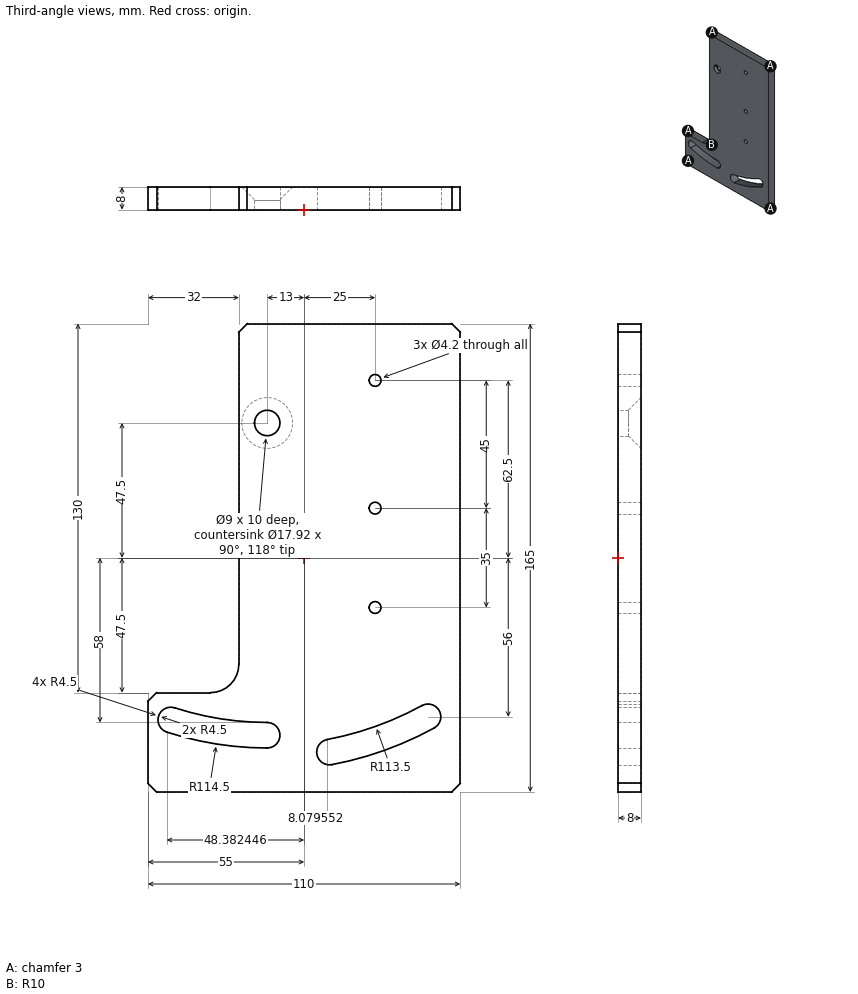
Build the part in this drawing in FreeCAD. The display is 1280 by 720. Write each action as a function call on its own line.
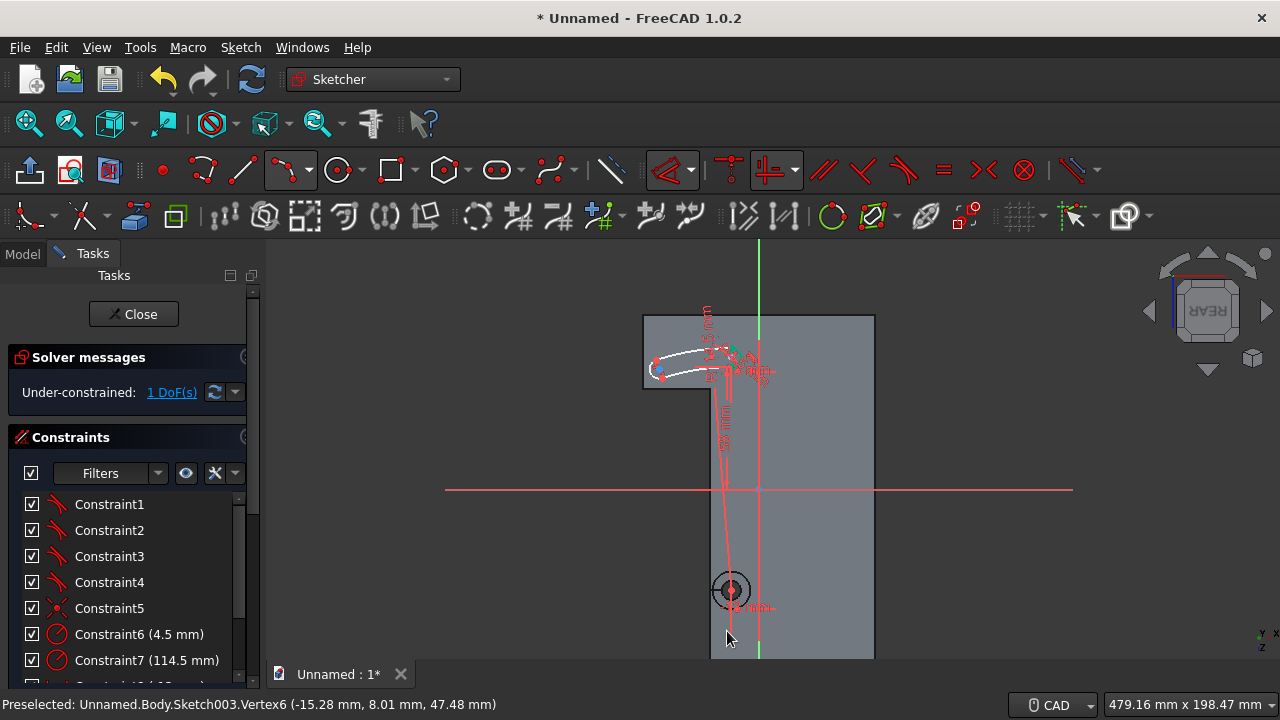
scroll(705, 383, up, 3)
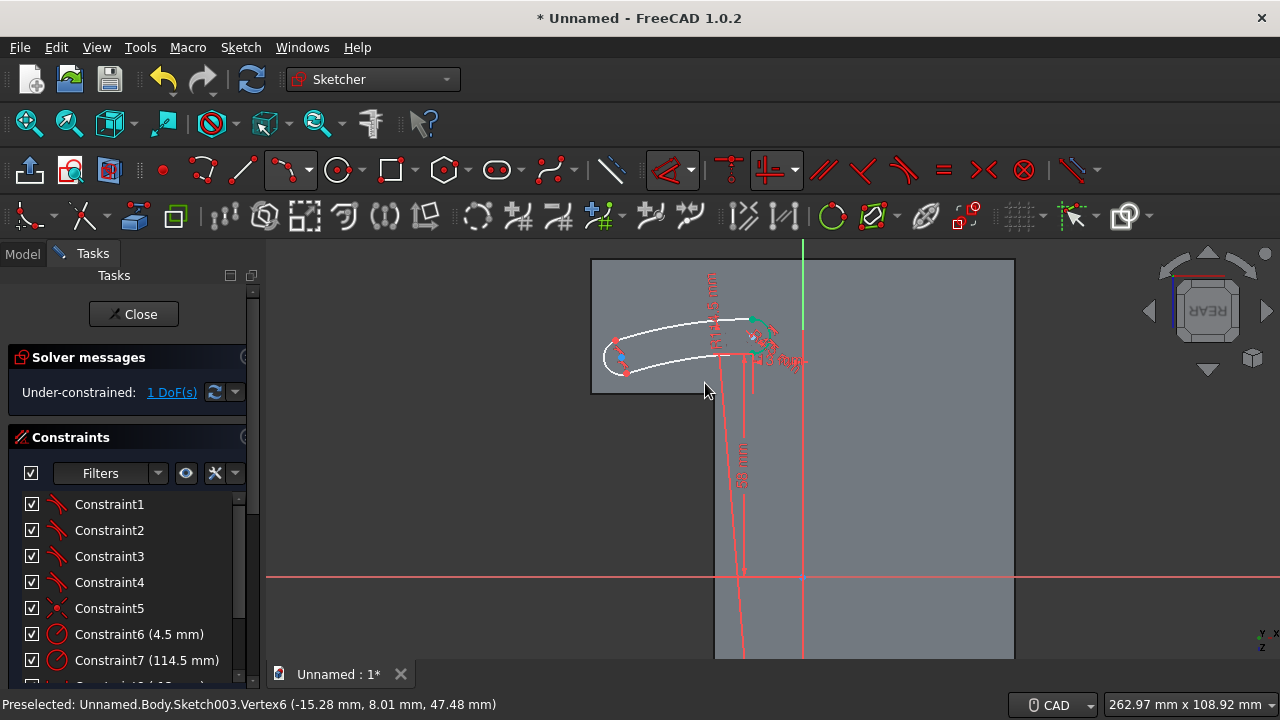
click(616, 341)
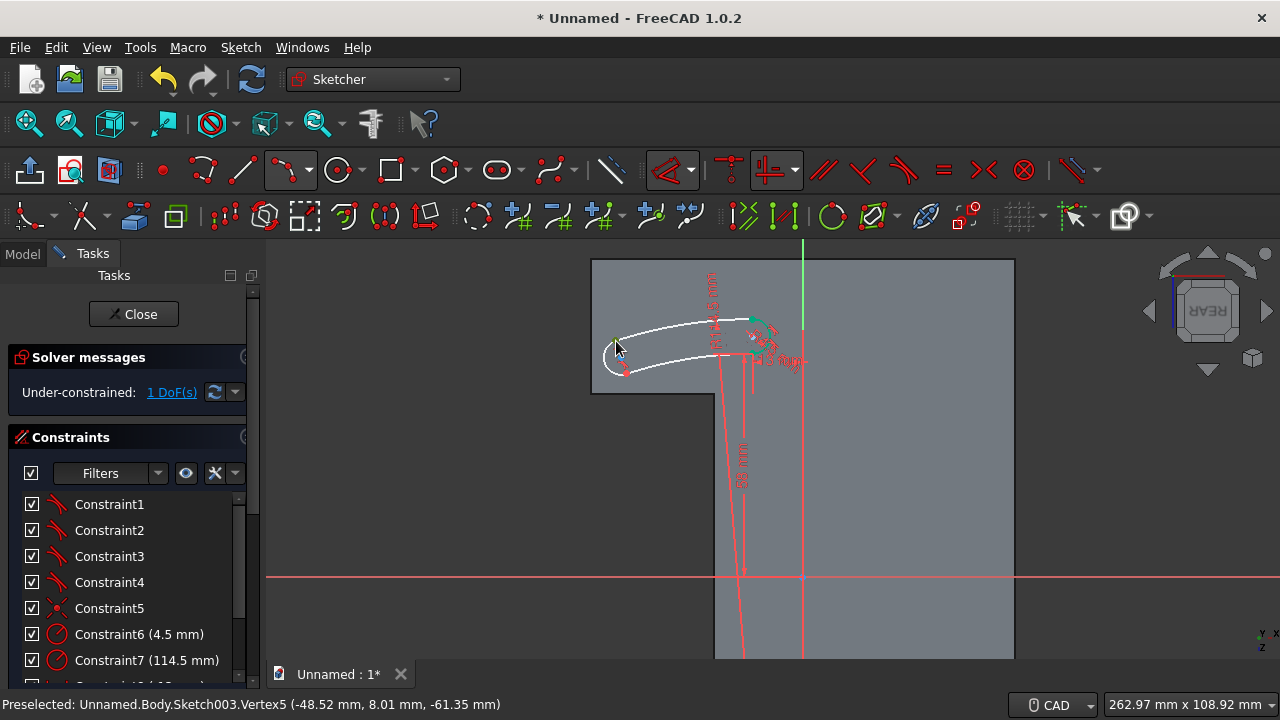
key(l)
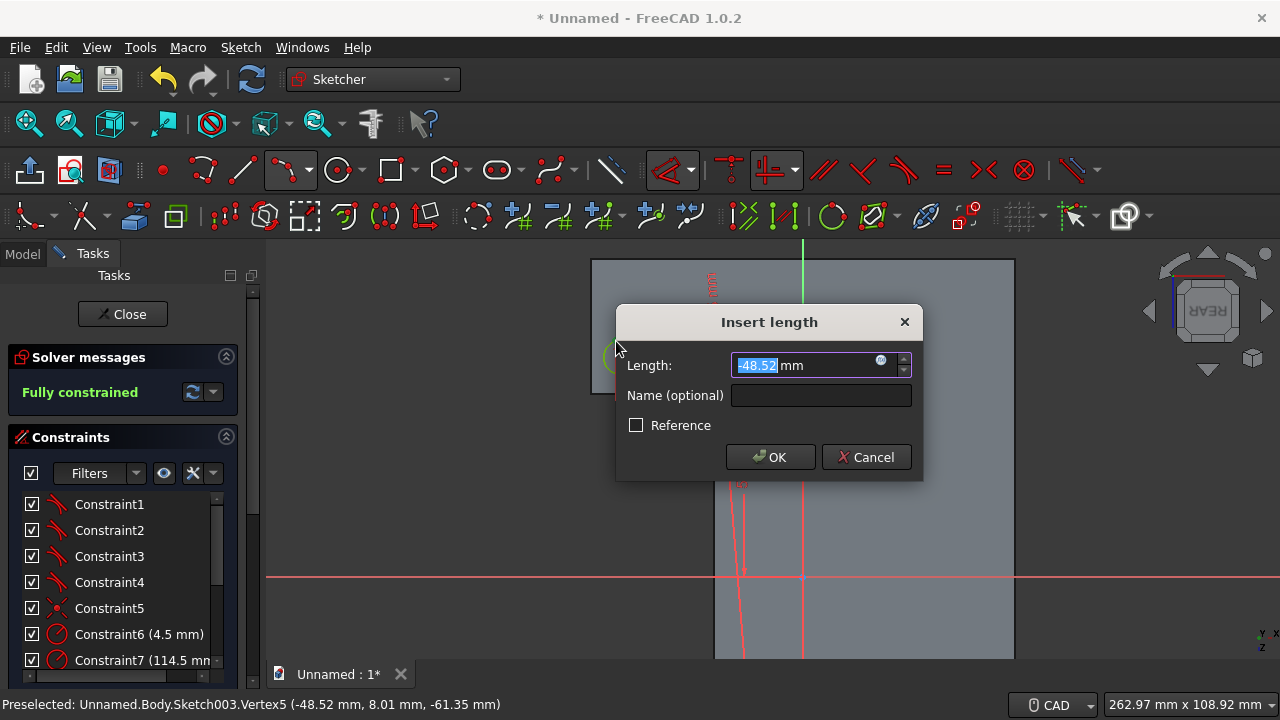
text(-48.382446)
key(Return)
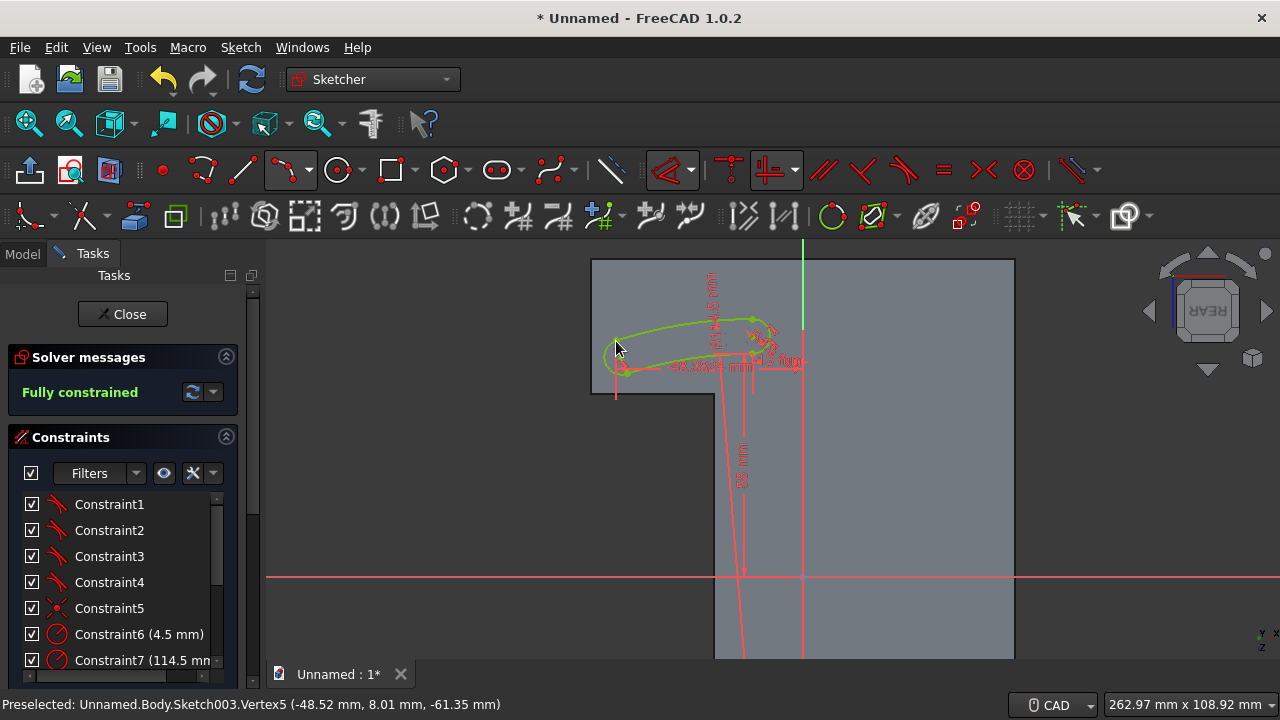
click(123, 314)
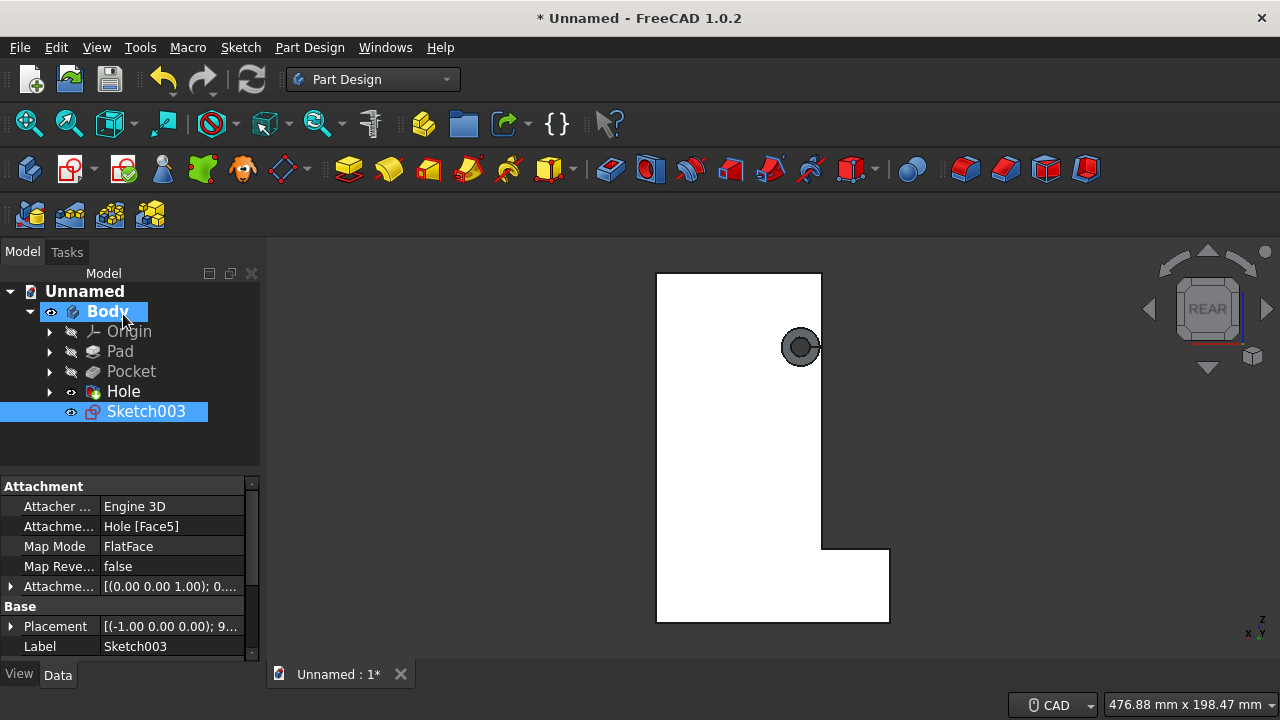
click(612, 170)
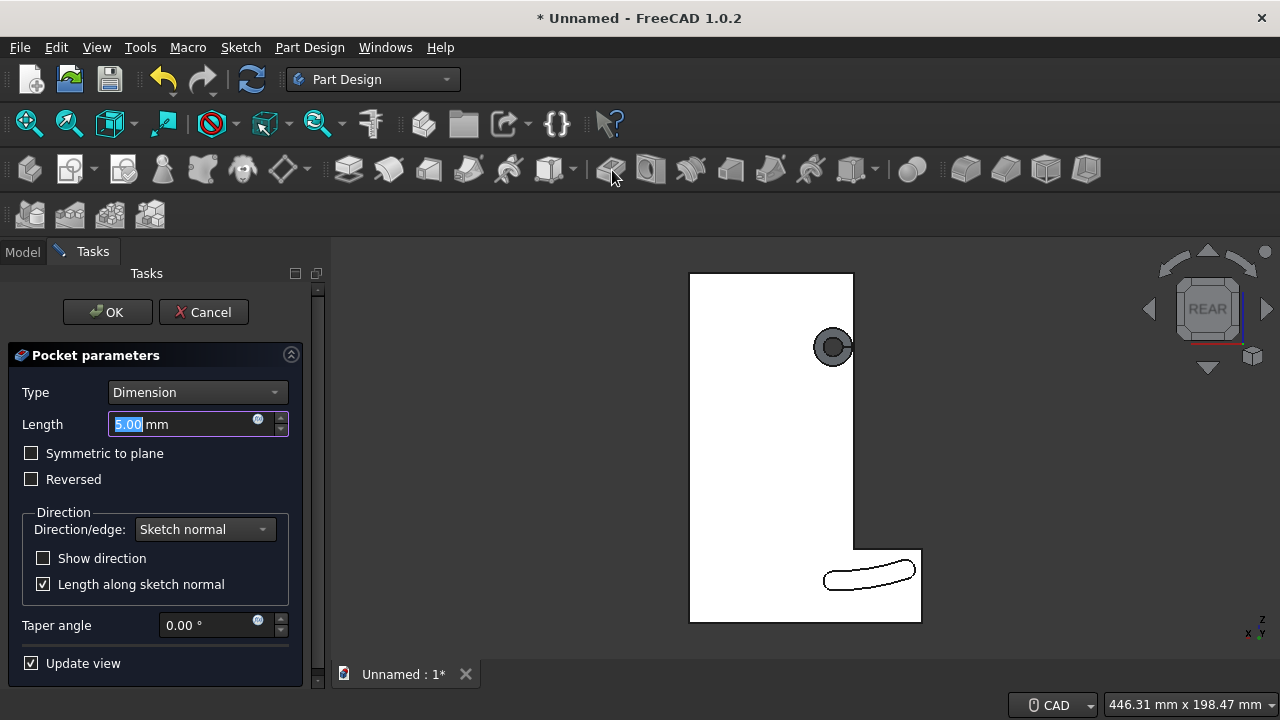
text(8)
key(Tab)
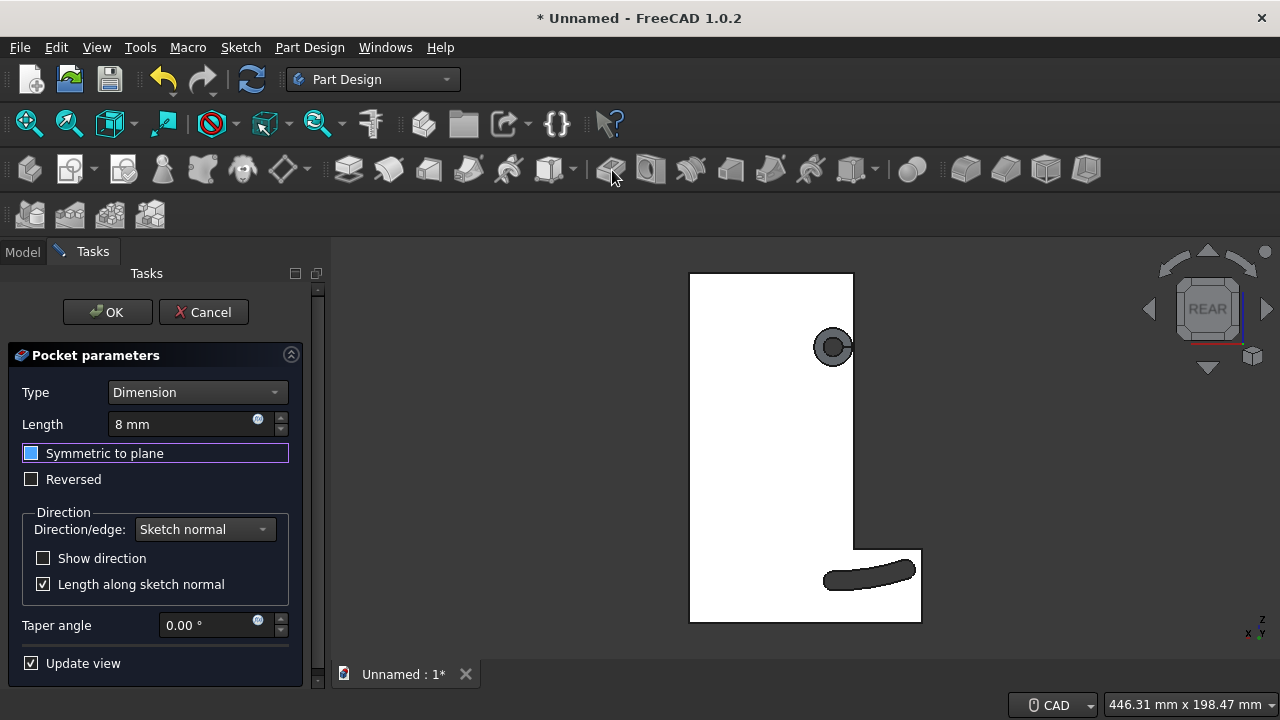
click(108, 312)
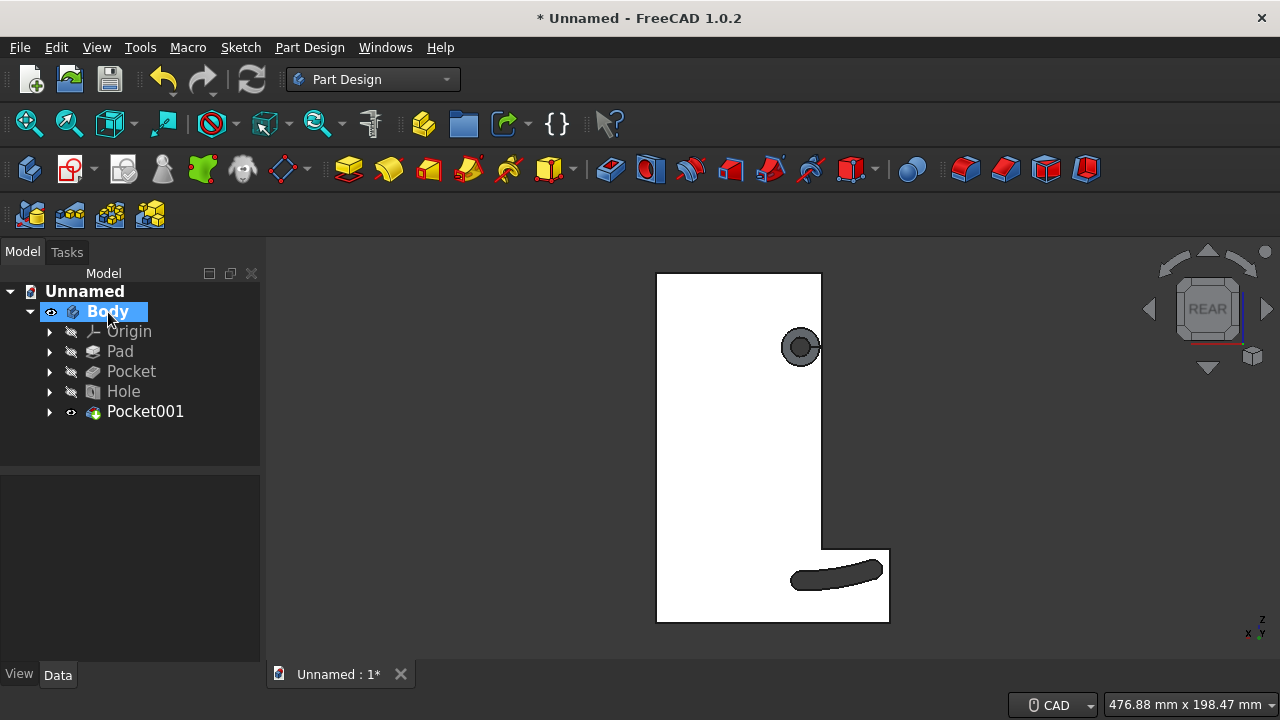
click(740, 447)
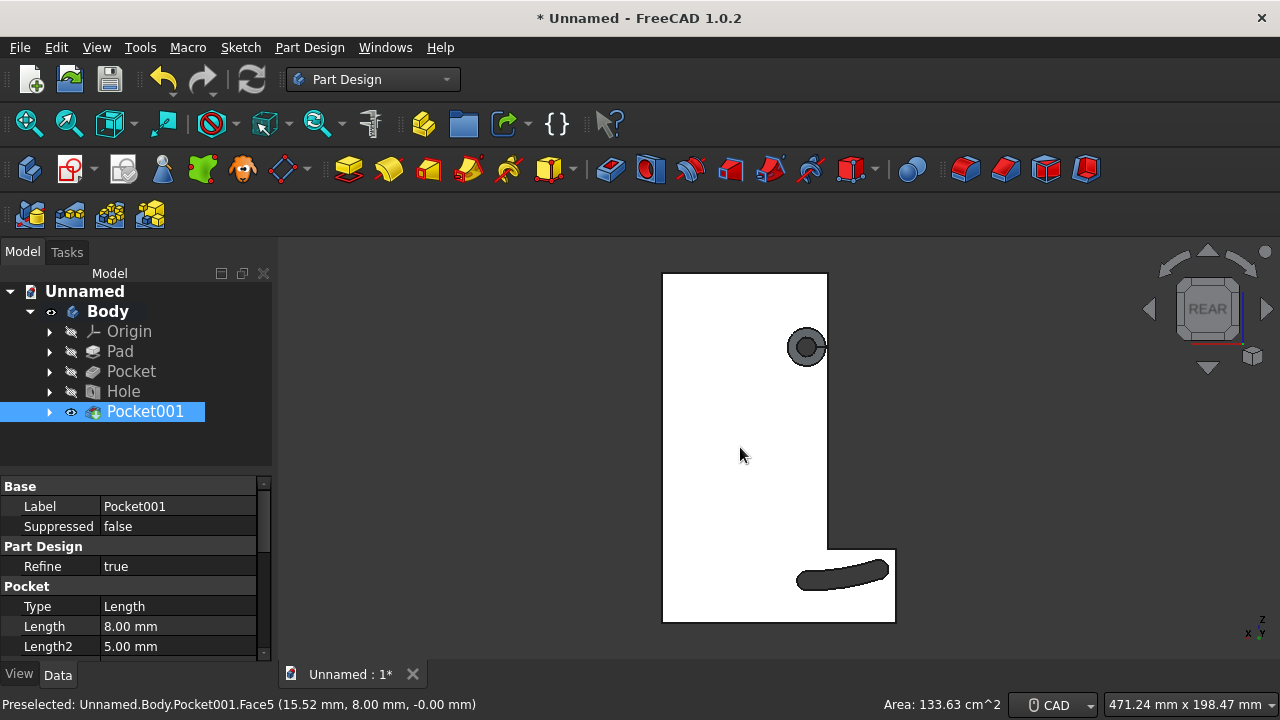
click(70, 170)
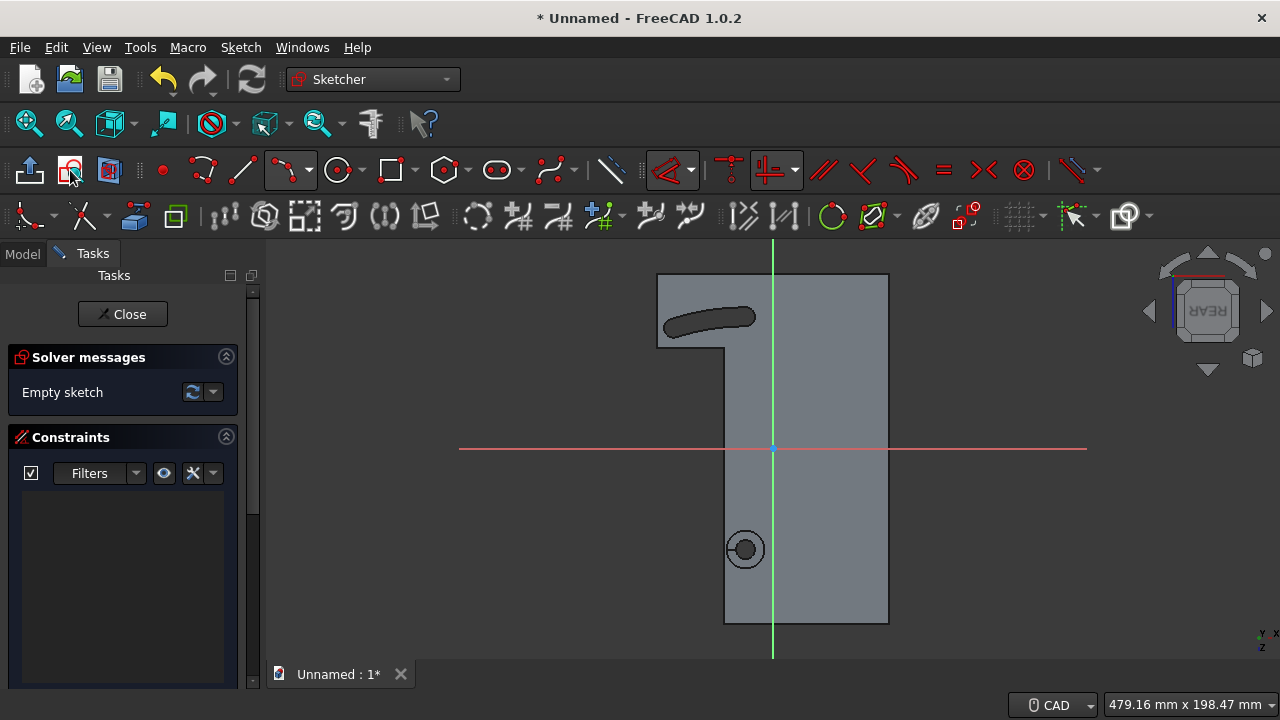
scroll(848, 278, up, 3)